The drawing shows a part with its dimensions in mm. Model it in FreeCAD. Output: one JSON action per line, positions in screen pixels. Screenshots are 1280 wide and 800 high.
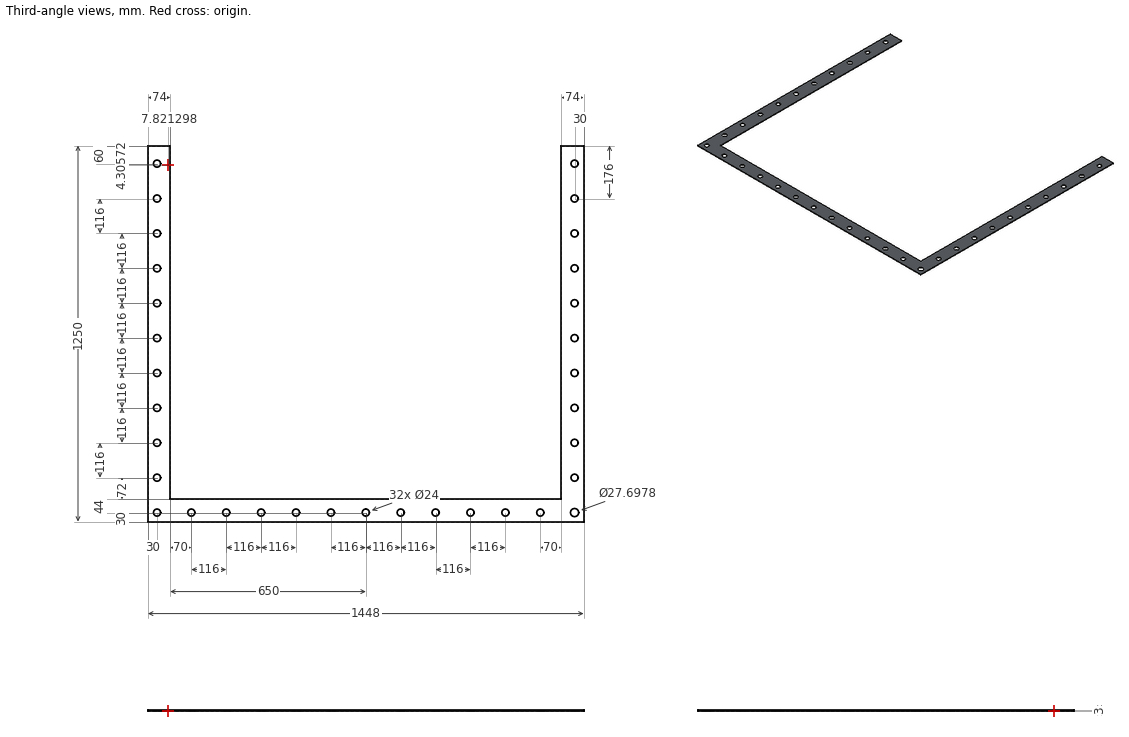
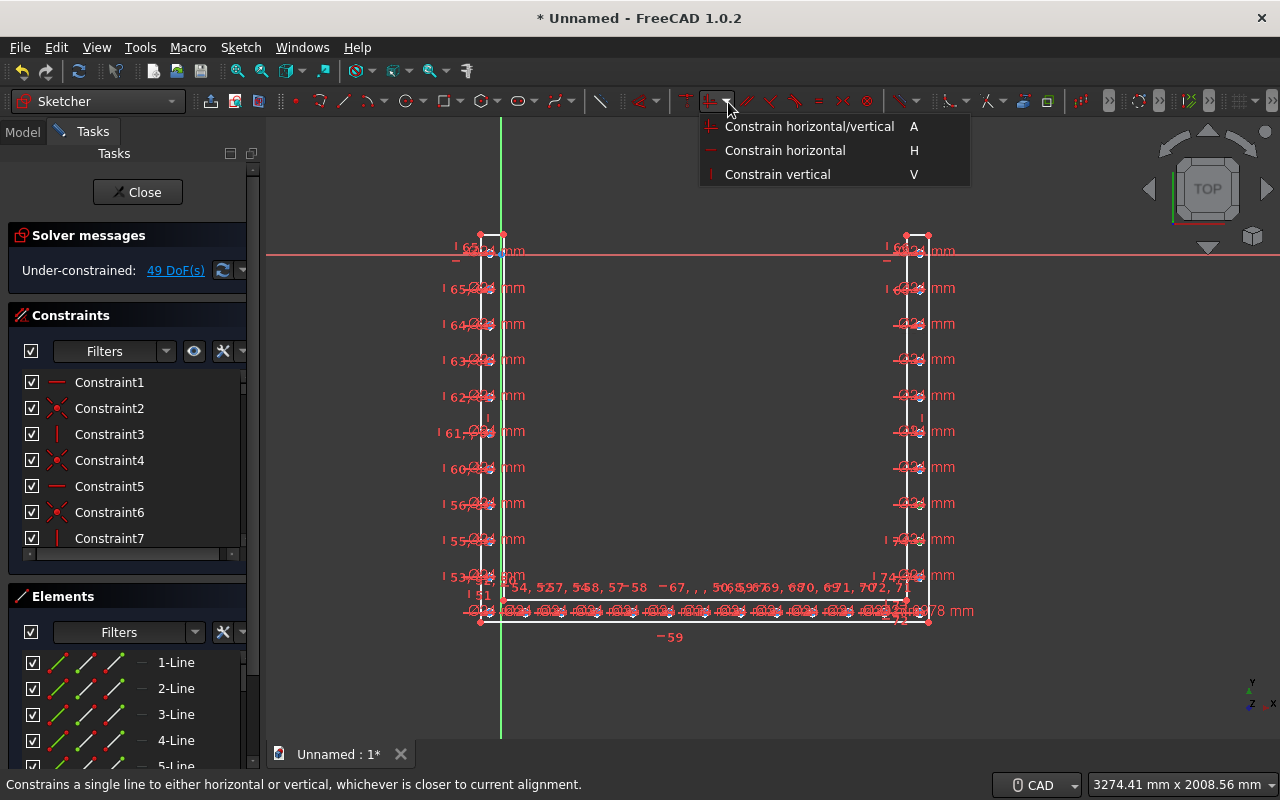
{"action": "left_click", "coordinate": [835, 174]}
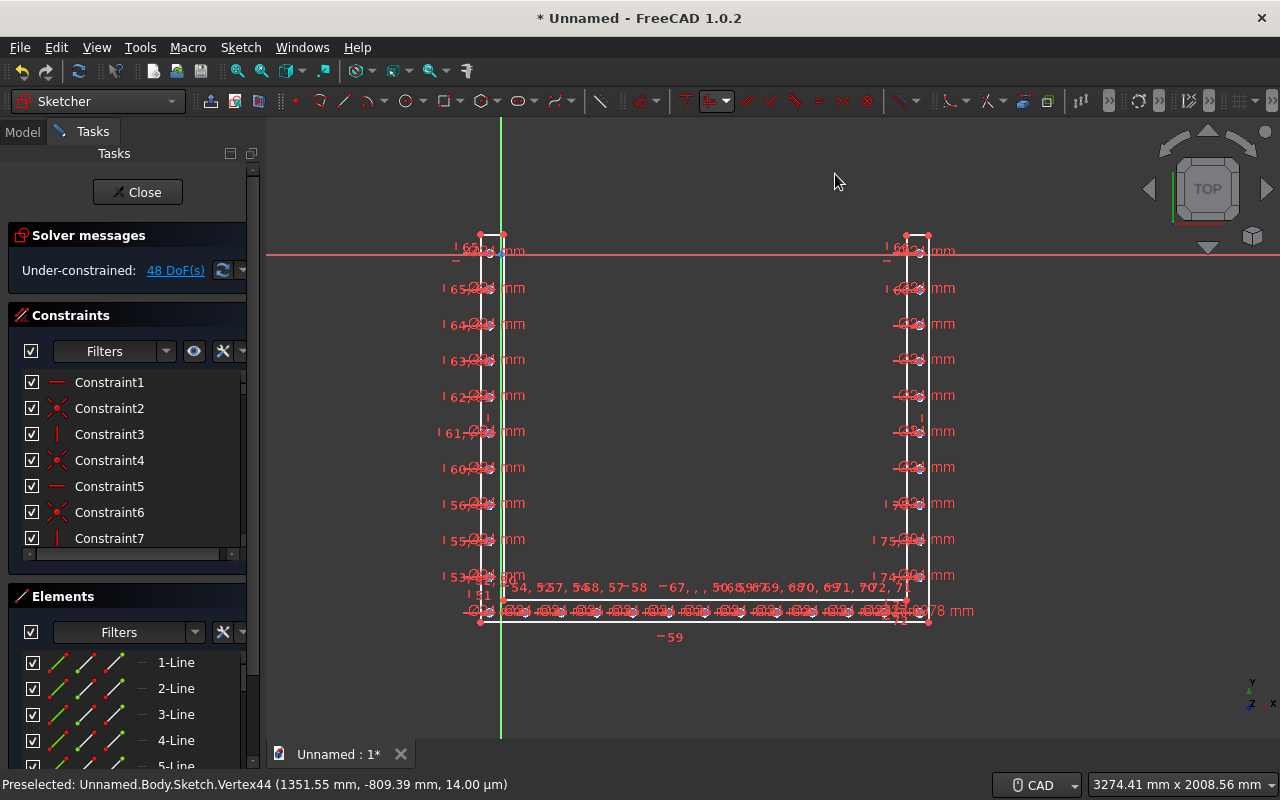
{"action": "left_click", "coordinate": [920, 505]}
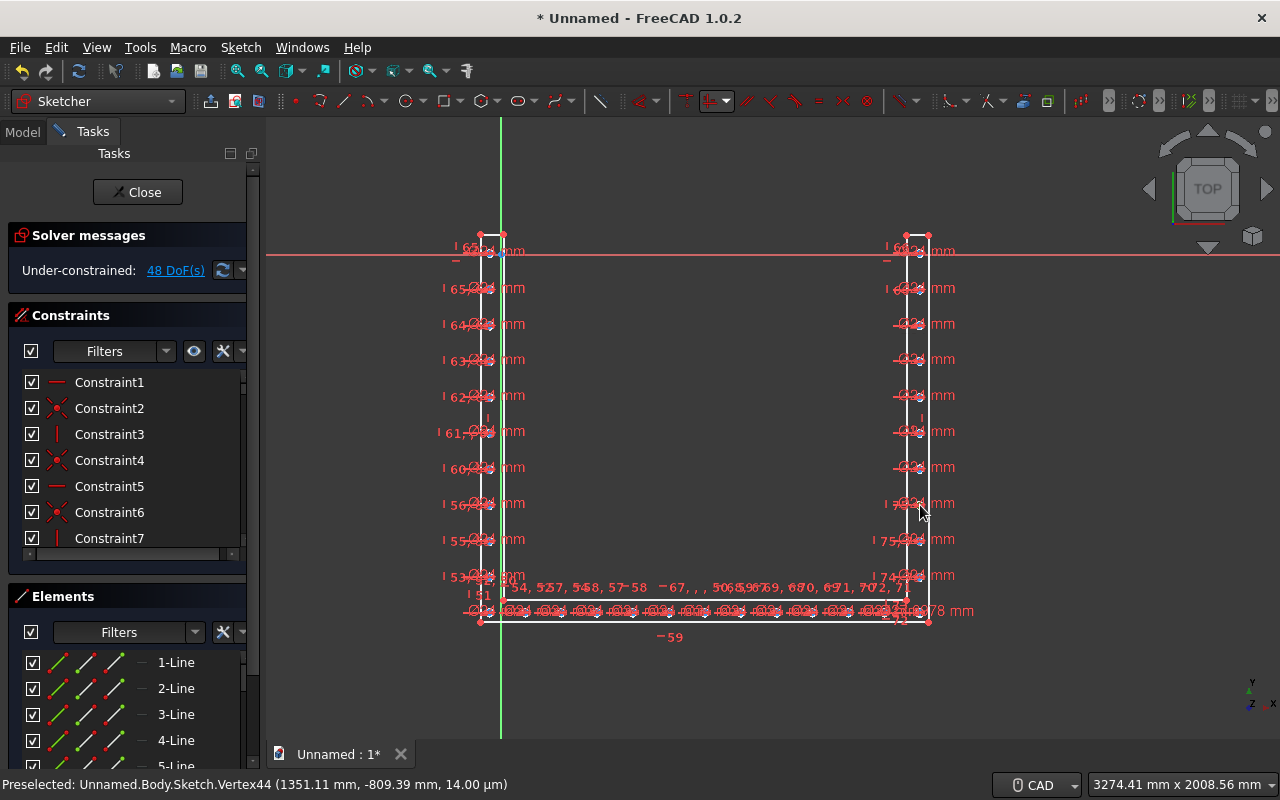
{"action": "left_click", "coordinate": [920, 469]}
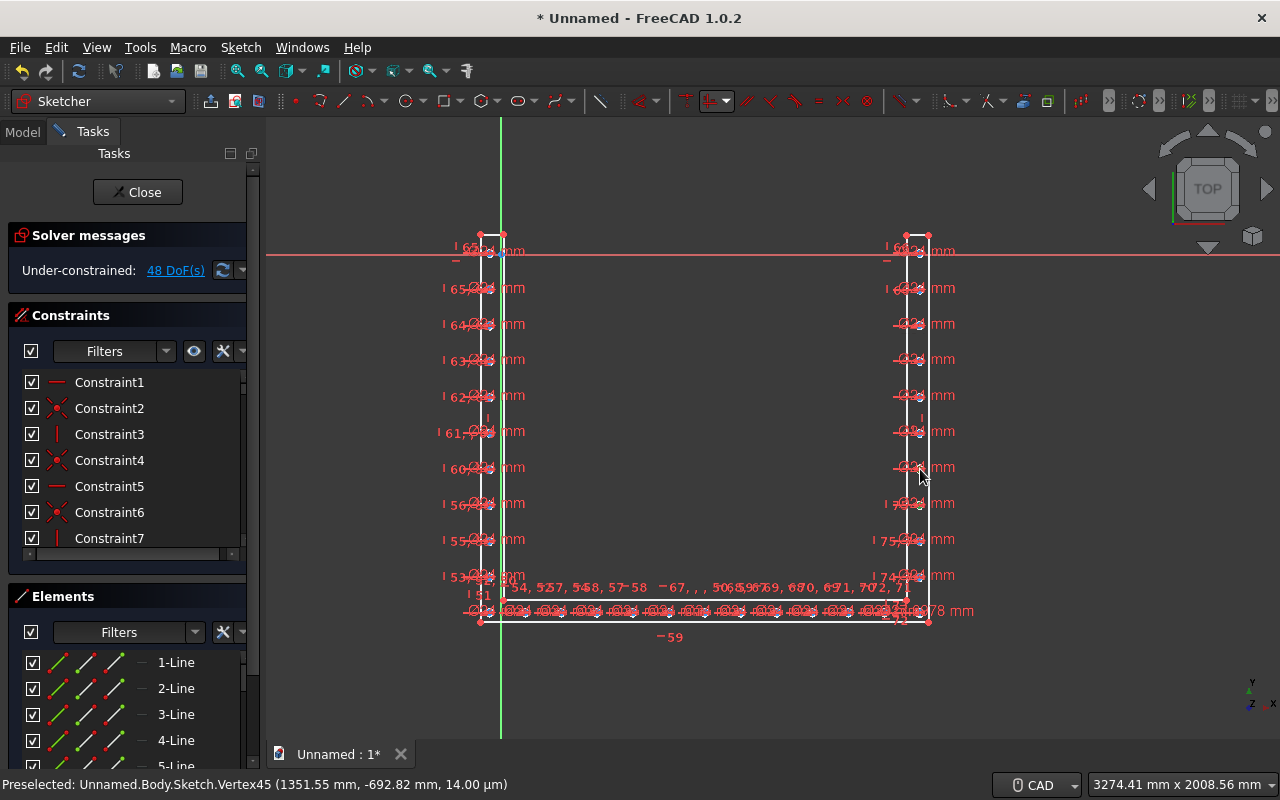
{"action": "left_click", "coordinate": [728, 102]}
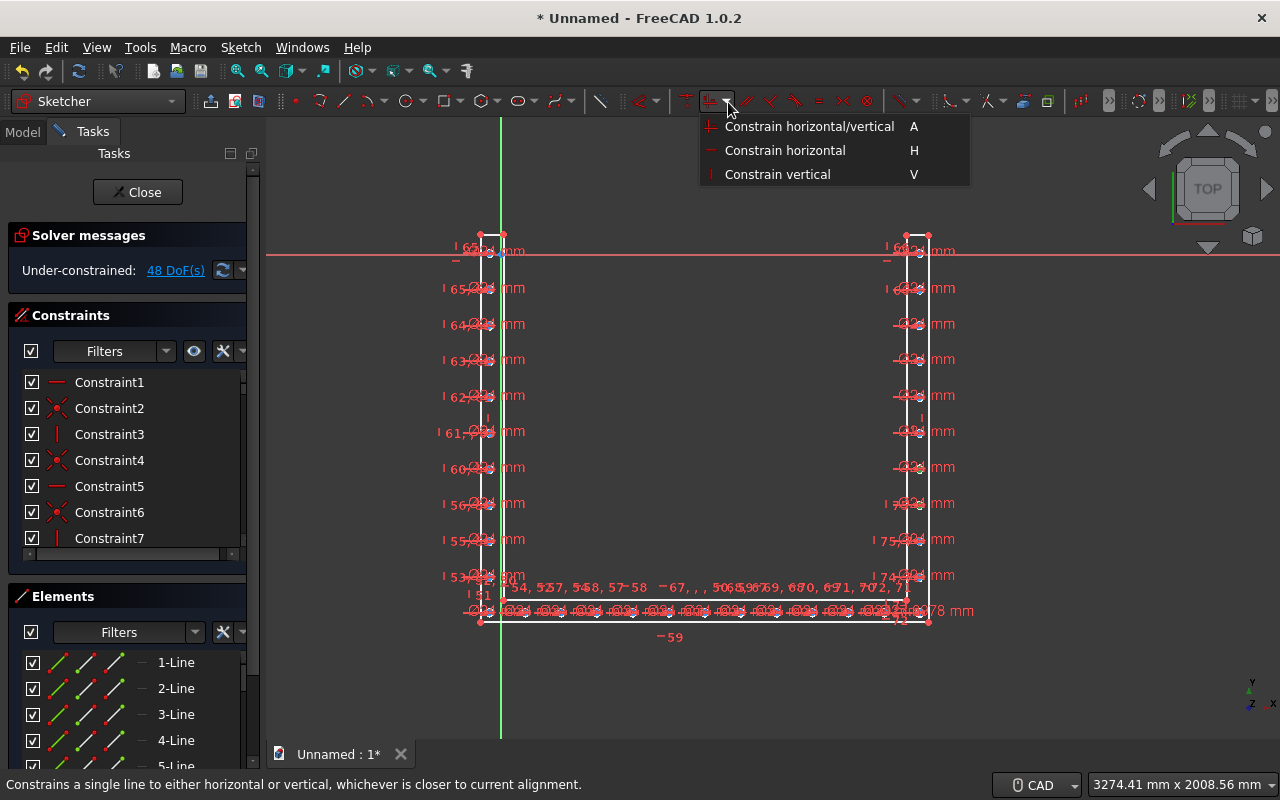
{"action": "left_click", "coordinate": [835, 174]}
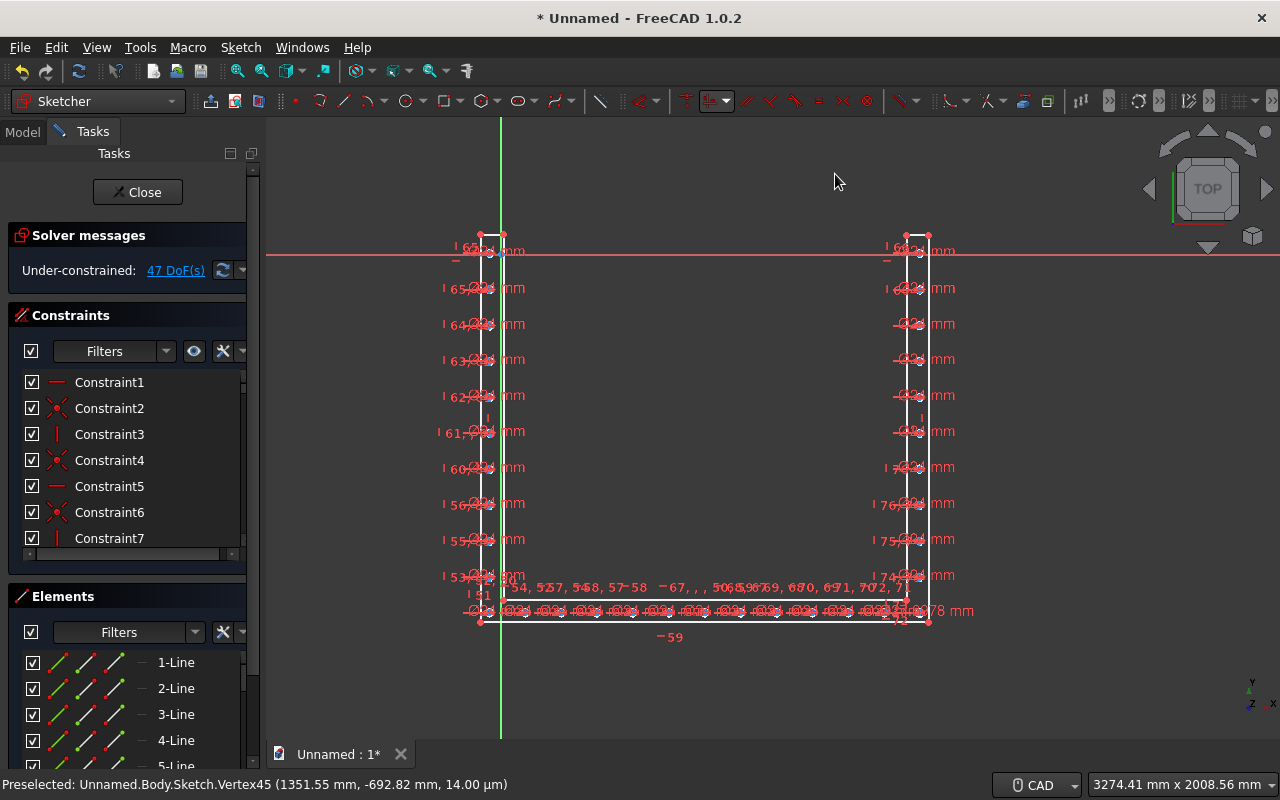
{"action": "left_click", "coordinate": [920, 469]}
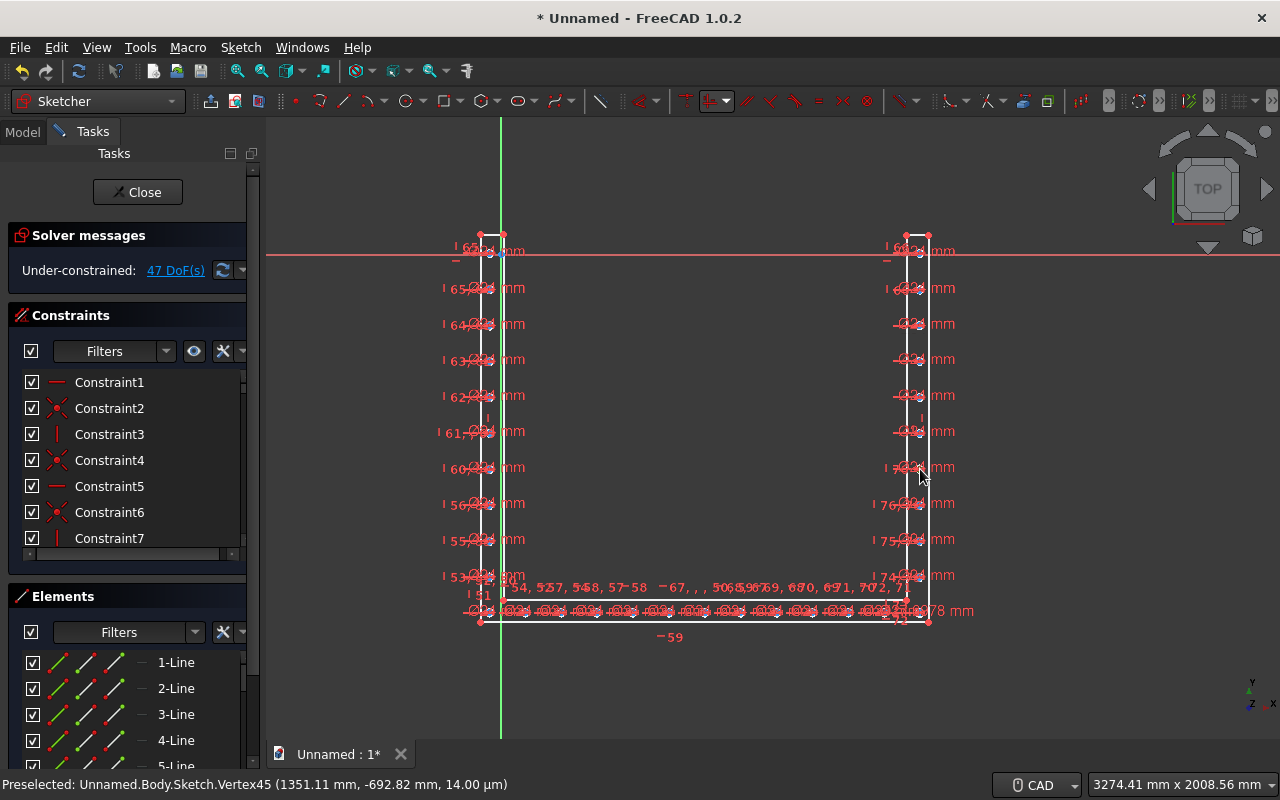
{"action": "left_click", "coordinate": [920, 433]}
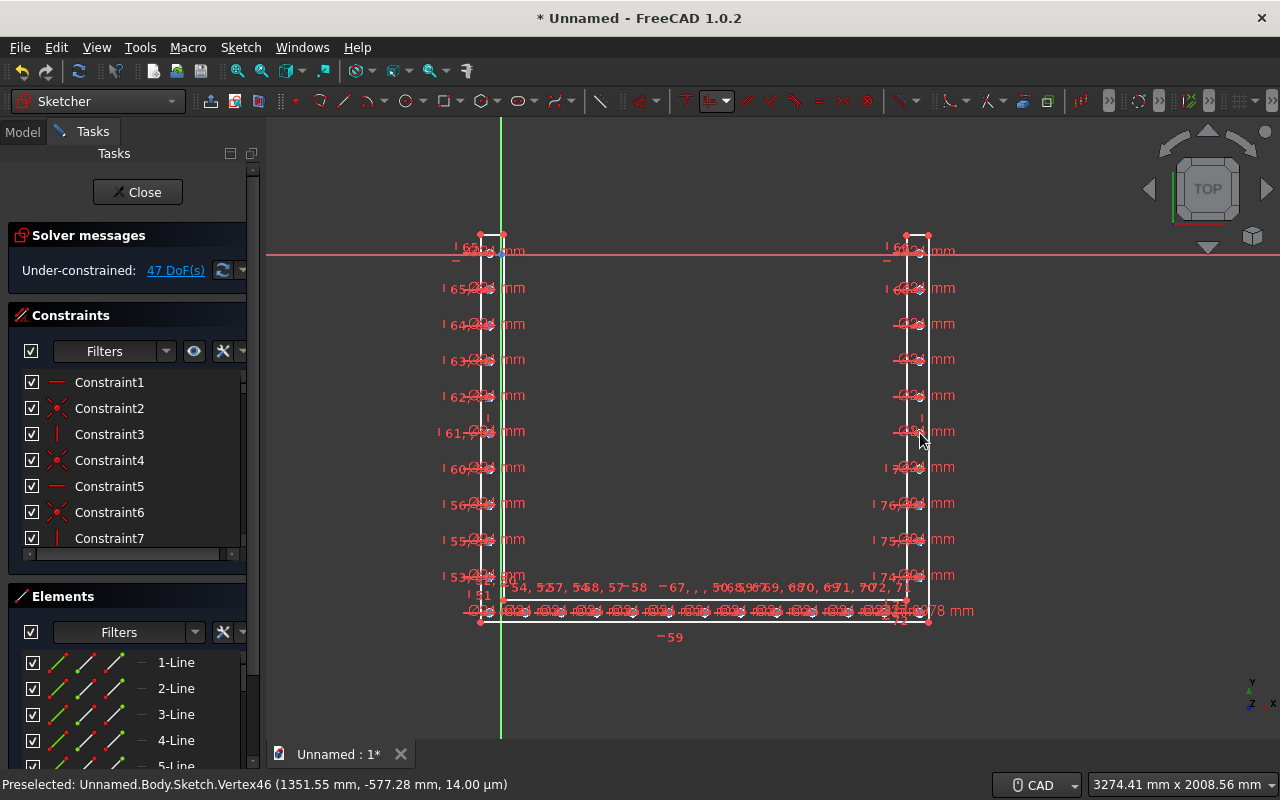
{"action": "left_click", "coordinate": [728, 102]}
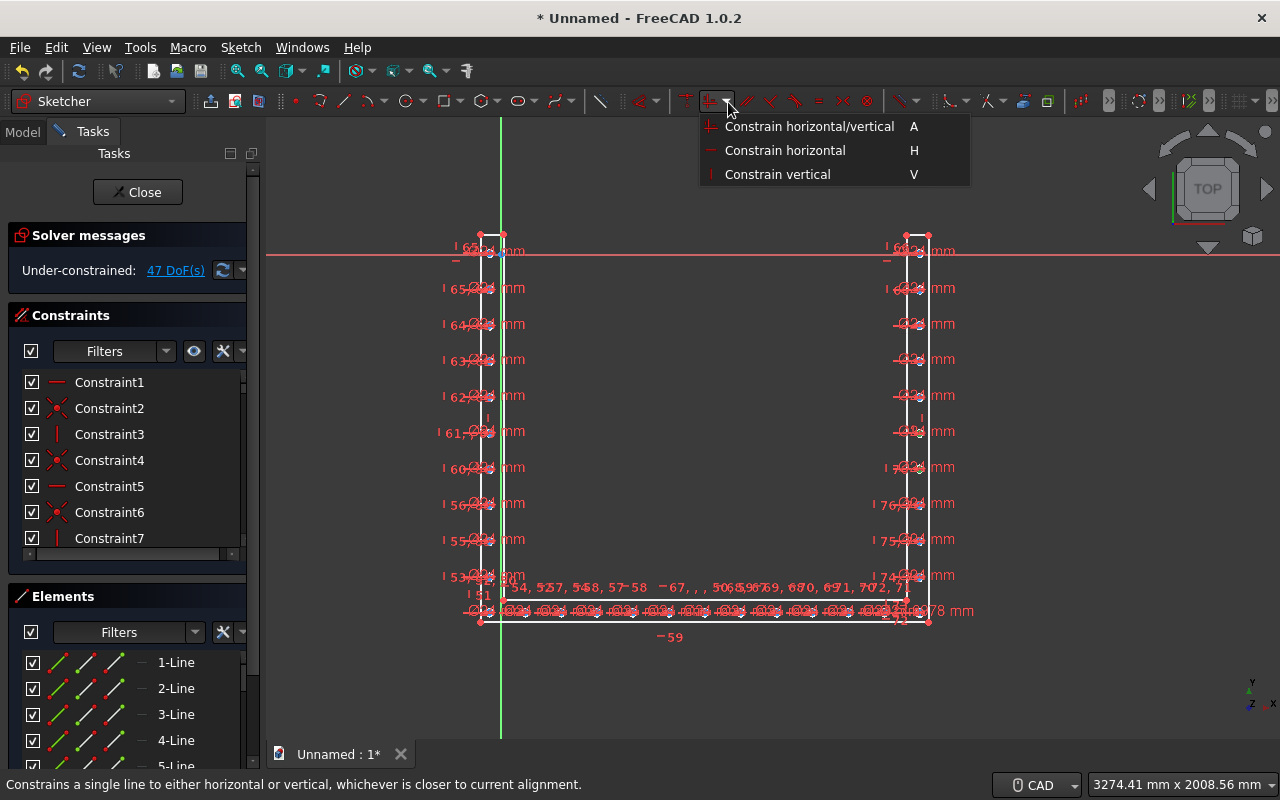
{"action": "left_click", "coordinate": [835, 174]}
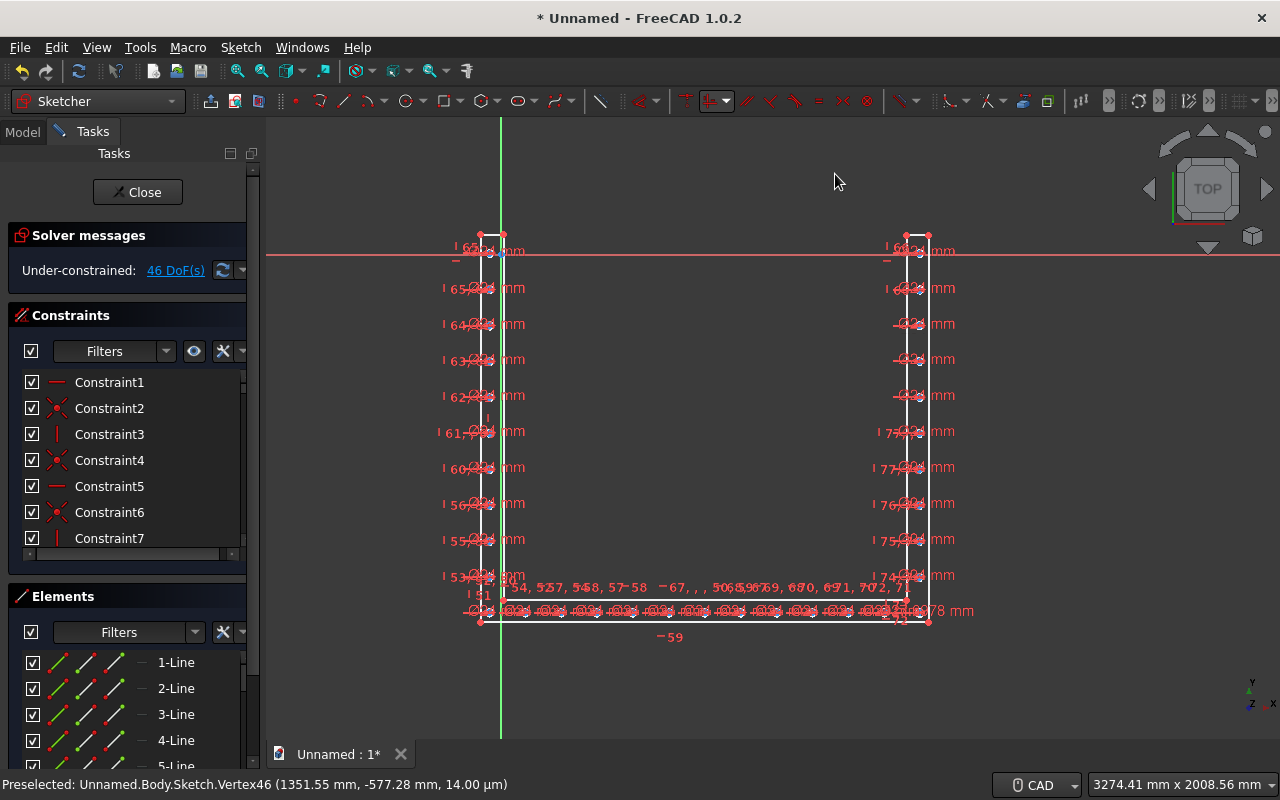
{"action": "left_click", "coordinate": [920, 290]}